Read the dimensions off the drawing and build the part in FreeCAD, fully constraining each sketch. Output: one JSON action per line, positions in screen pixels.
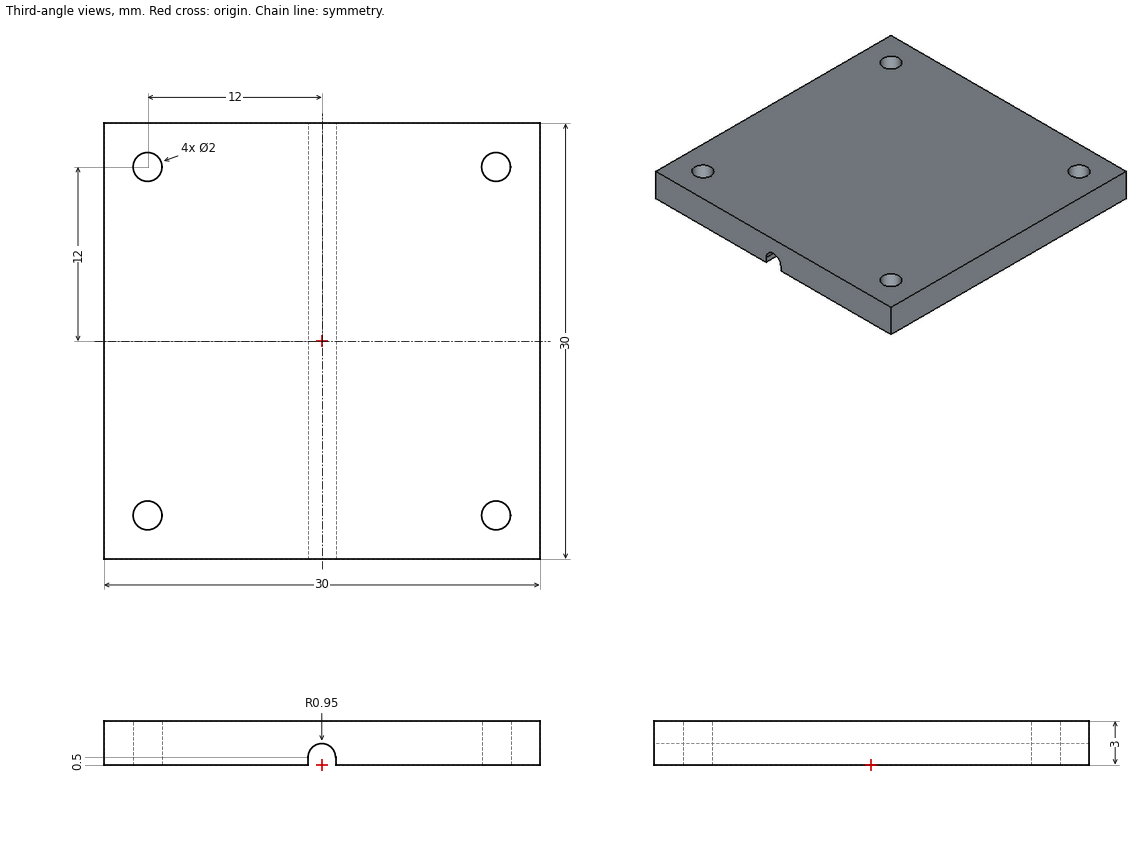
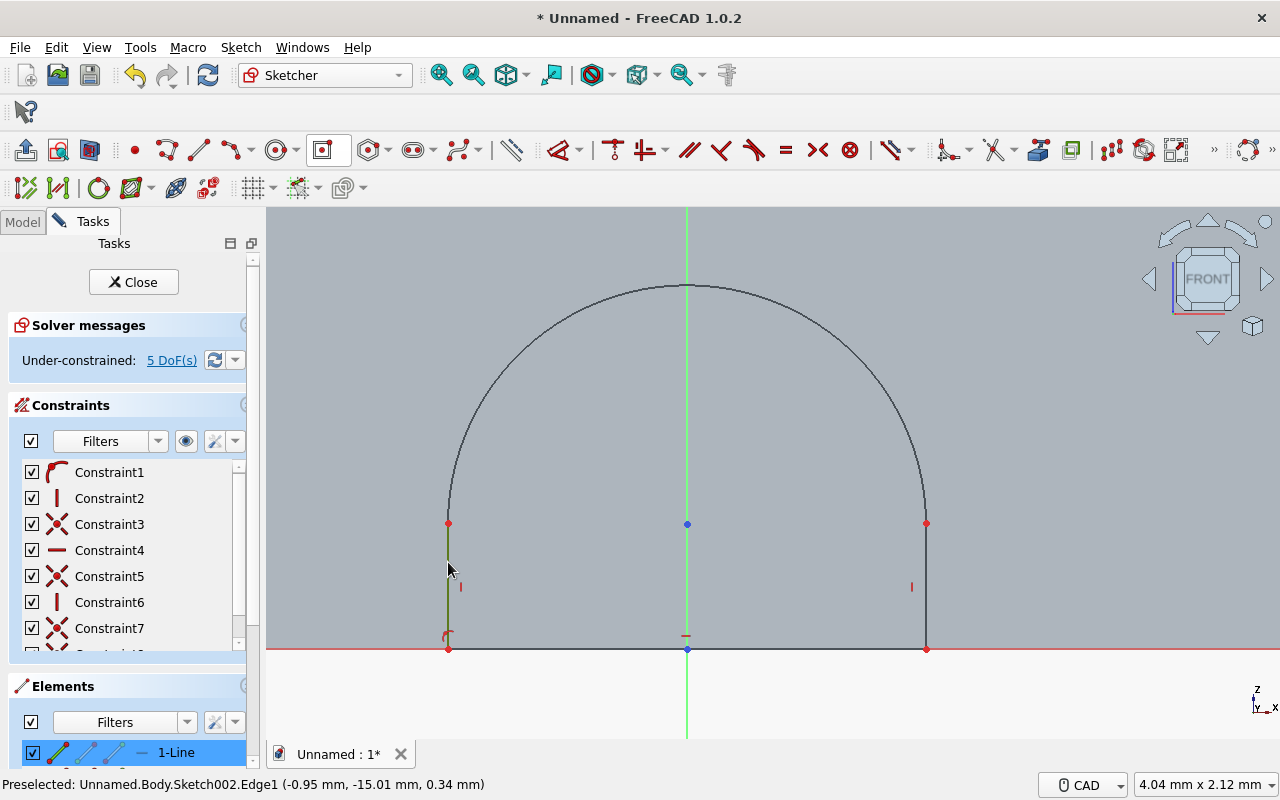
{"action": "left_click", "coordinate": [827, 331]}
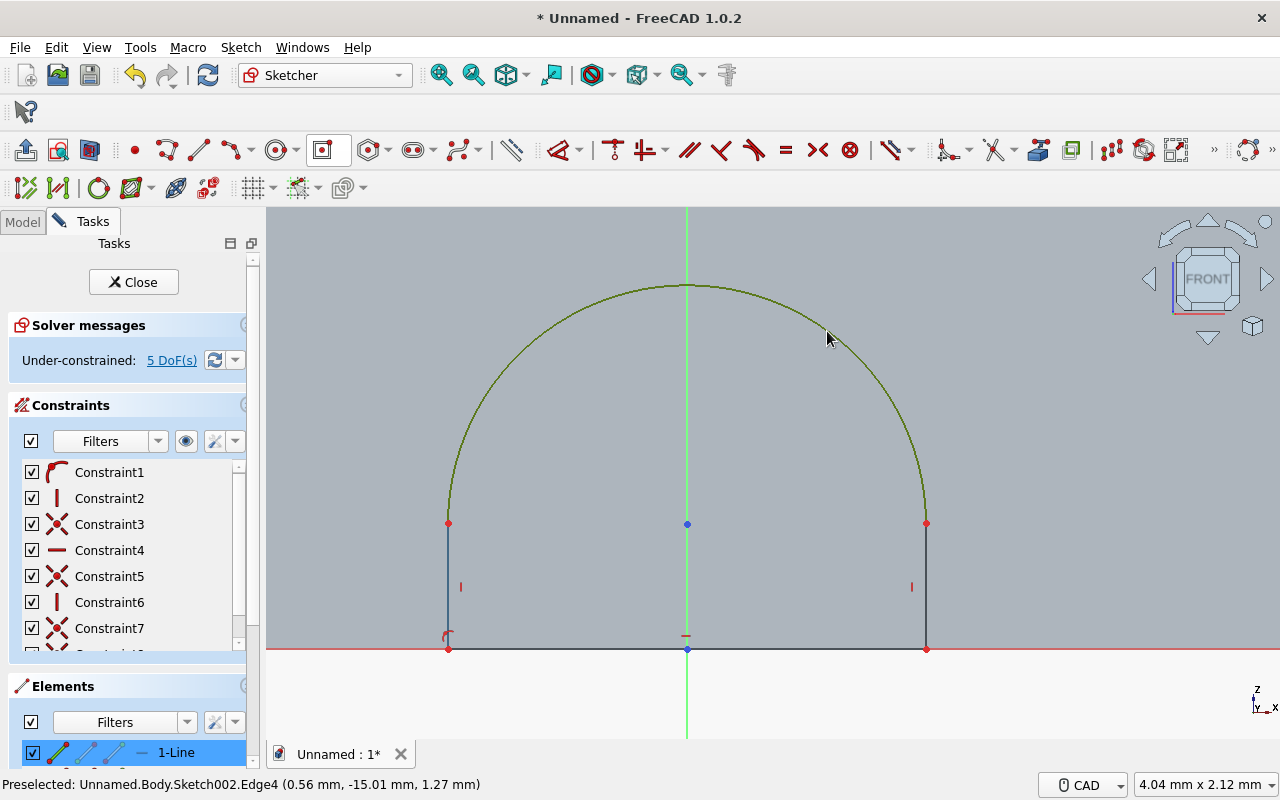
{"action": "left_click", "coordinate": [754, 150]}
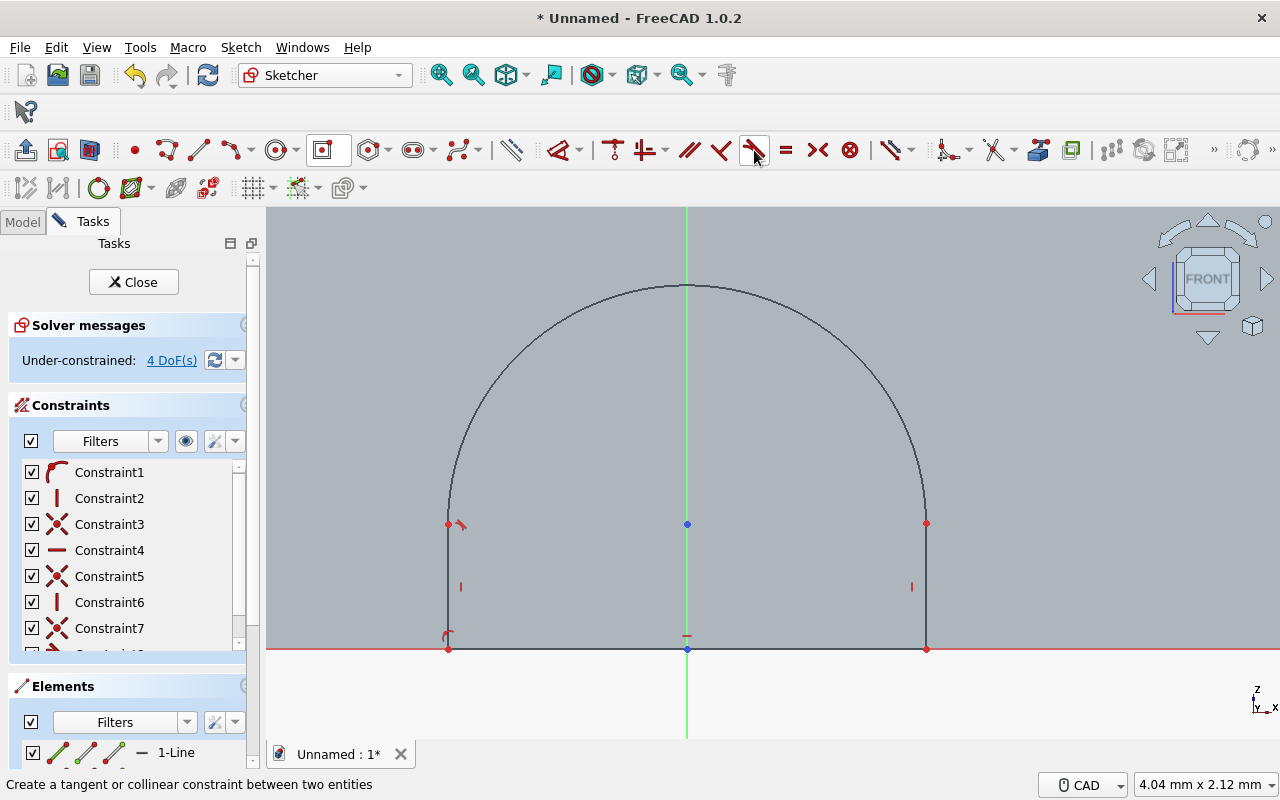
{"action": "left_click", "coordinate": [926, 612]}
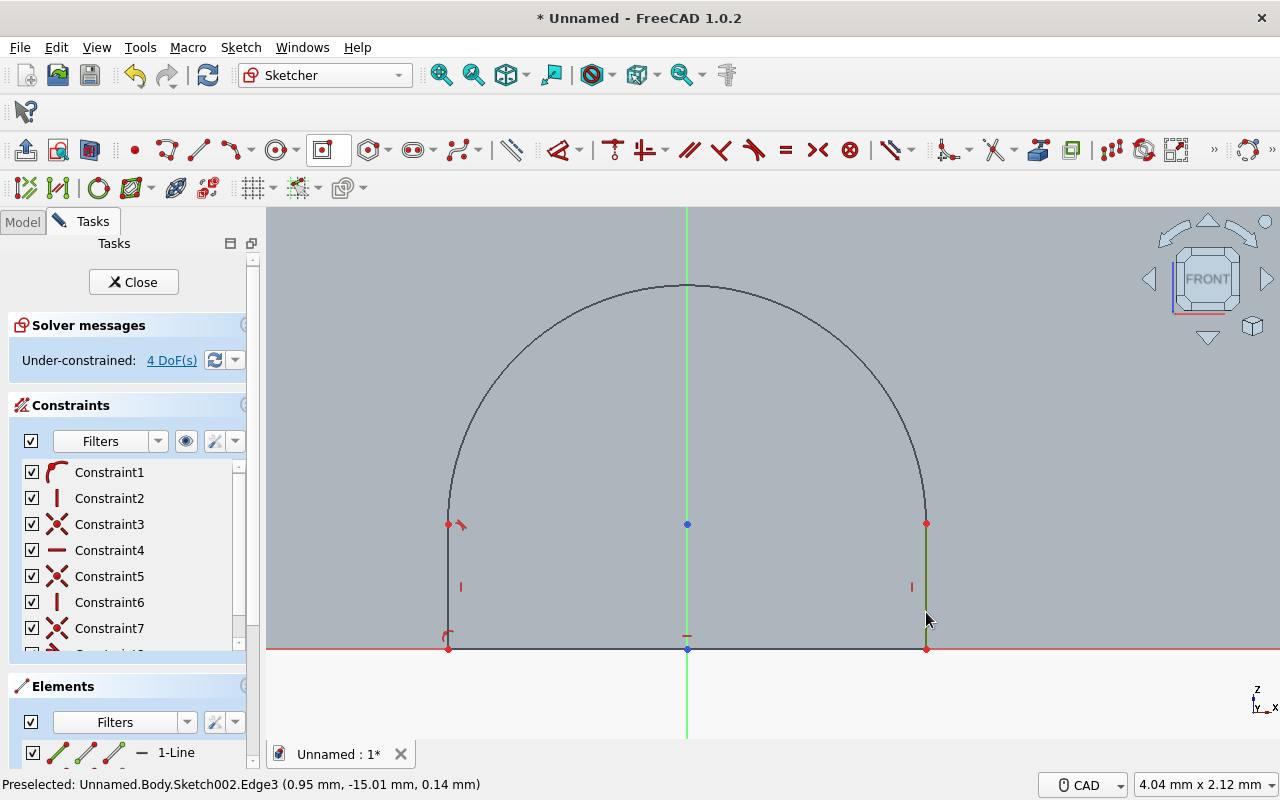
{"action": "left_click", "coordinate": [827, 331]}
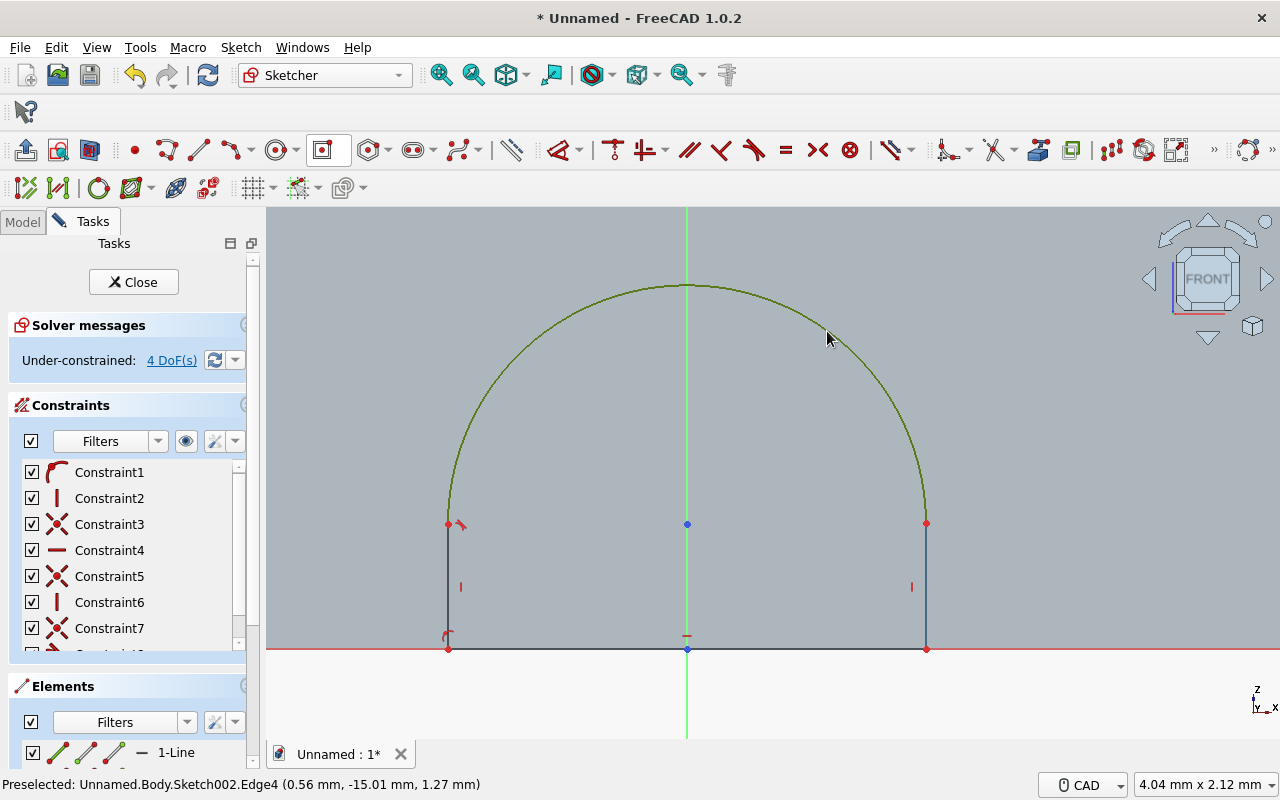
{"action": "left_click", "coordinate": [754, 150]}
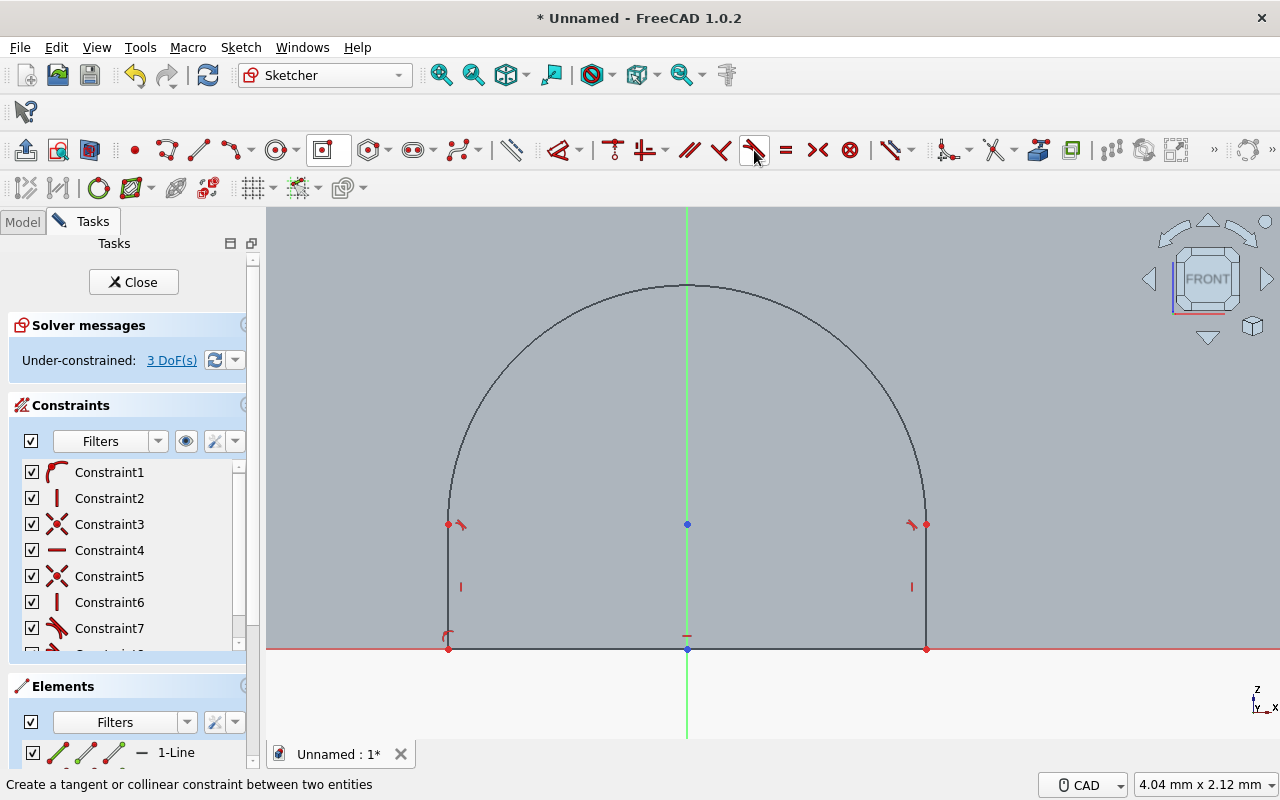
{"action": "left_click", "coordinate": [687, 524]}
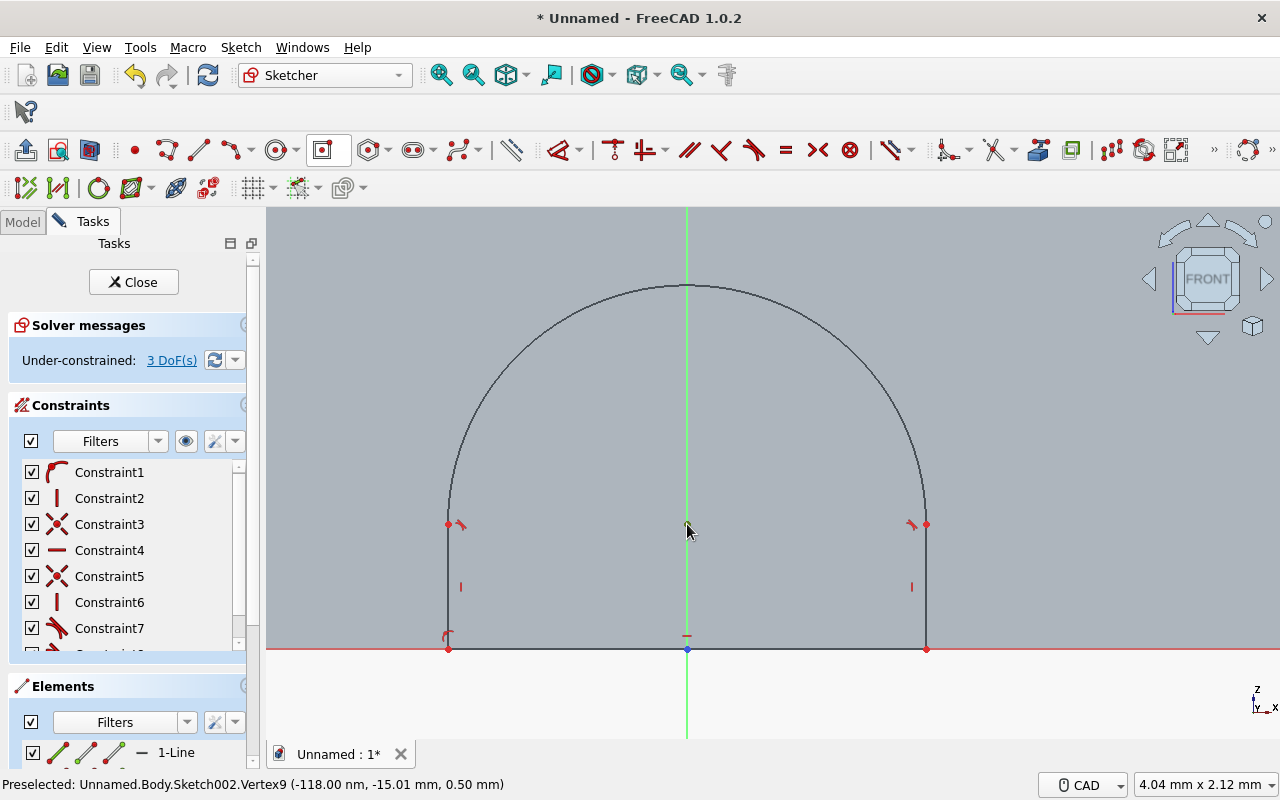
{"action": "left_click", "coordinate": [687, 609]}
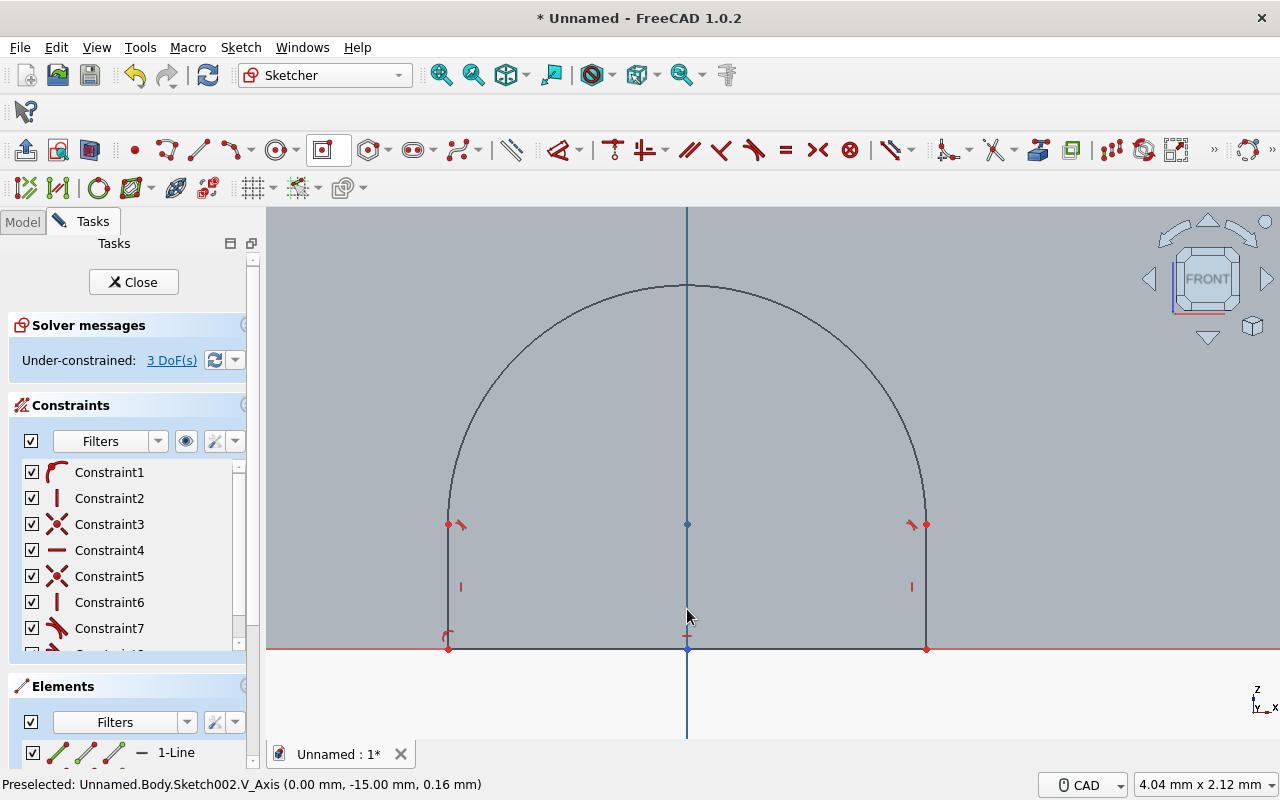
{"action": "left_click", "coordinate": [614, 150]}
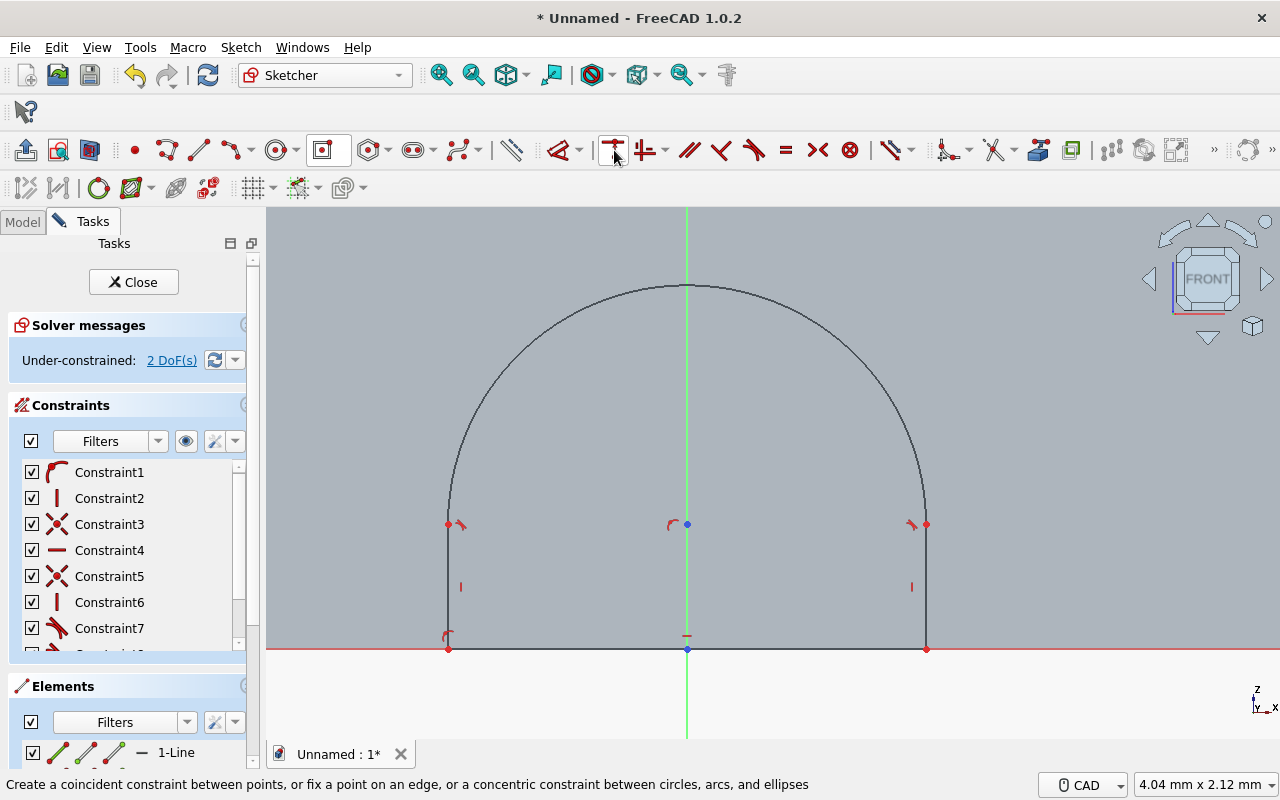
{"action": "key", "text": "d"}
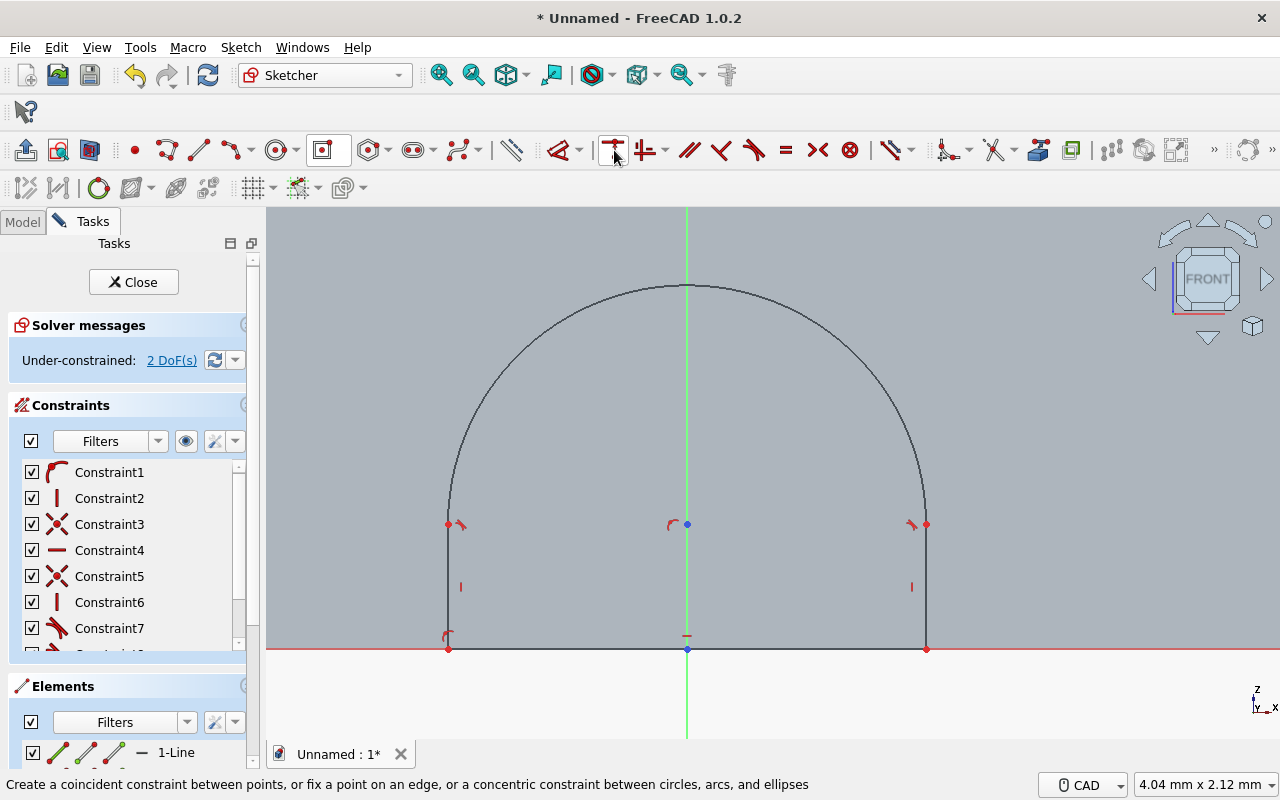
{"action": "left_click", "coordinate": [828, 331]}
{"action": "left_click", "coordinate": [847, 305]}